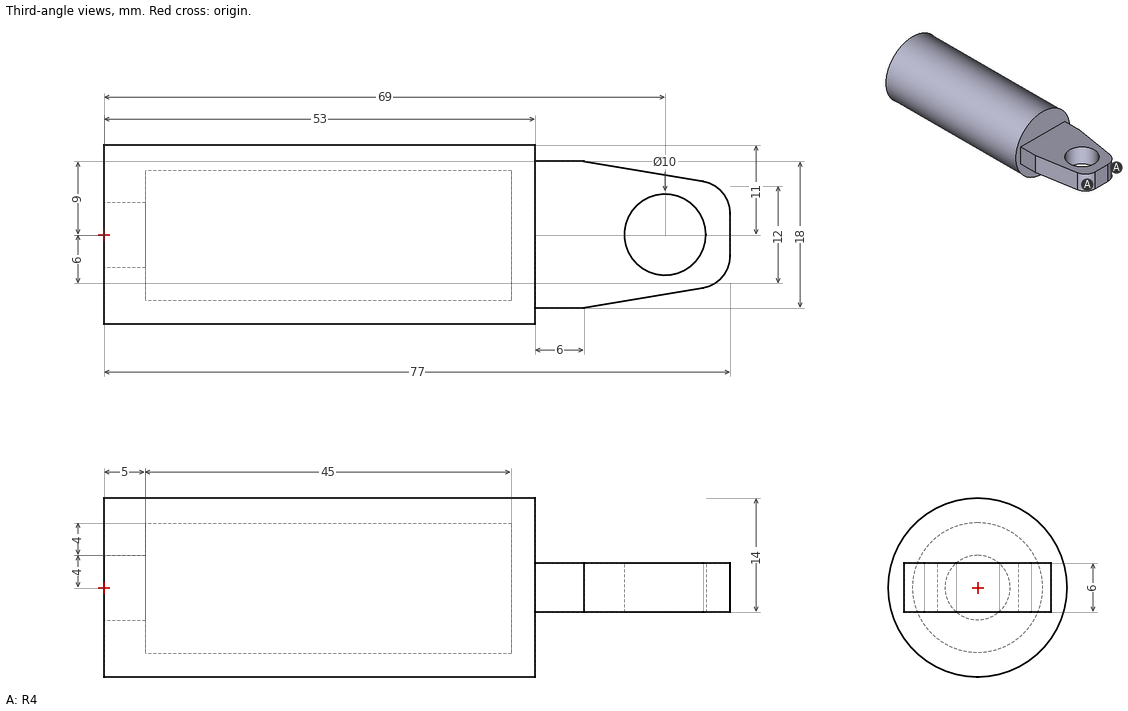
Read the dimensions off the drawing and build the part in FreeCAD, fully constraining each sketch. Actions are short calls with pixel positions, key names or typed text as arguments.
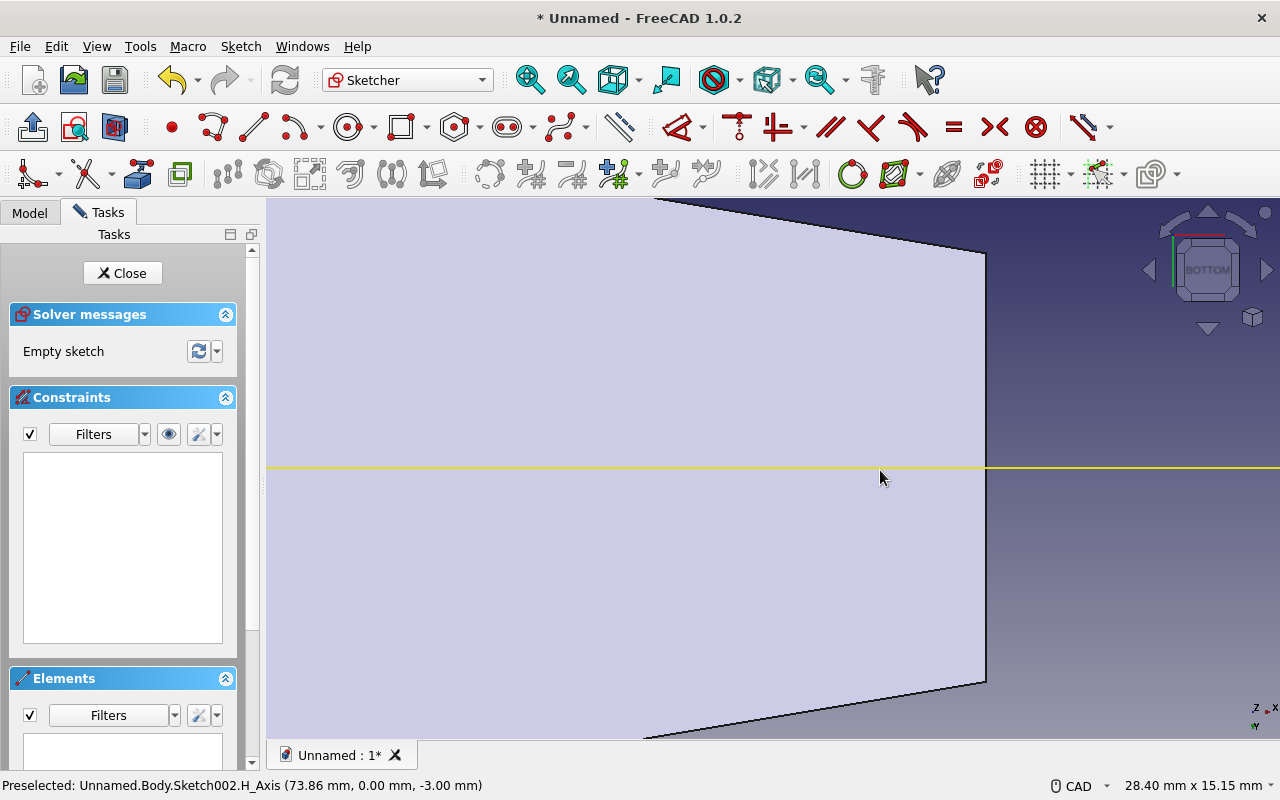
key(g)
key(c)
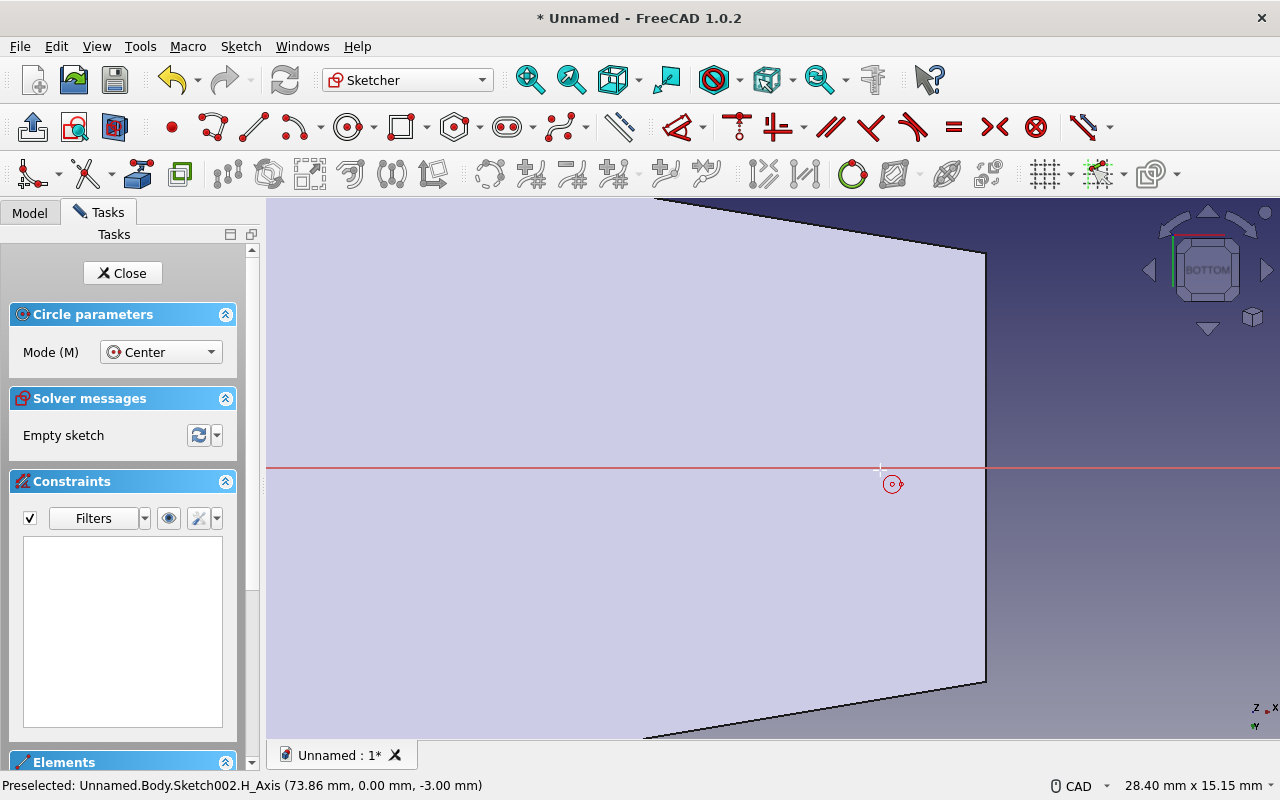
click(701, 468)
click(827, 341)
key(Escape)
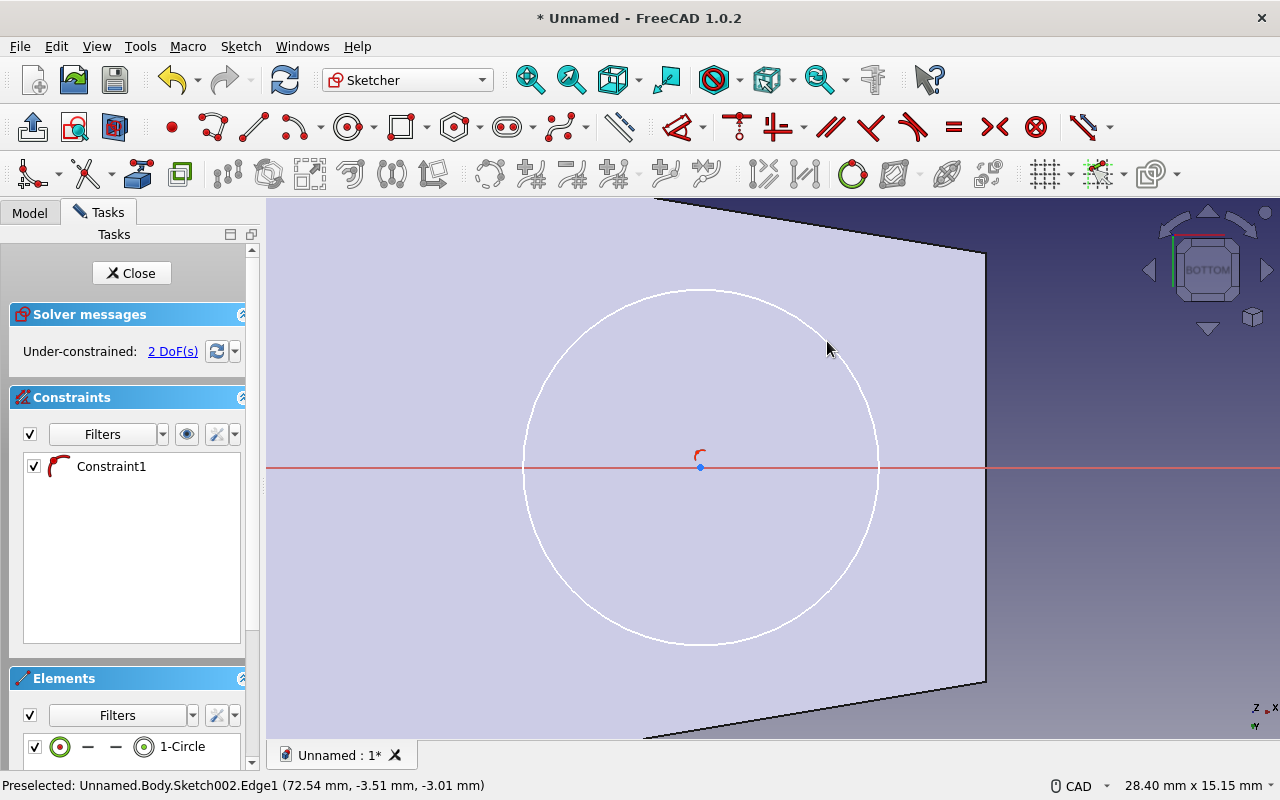
click(826, 341)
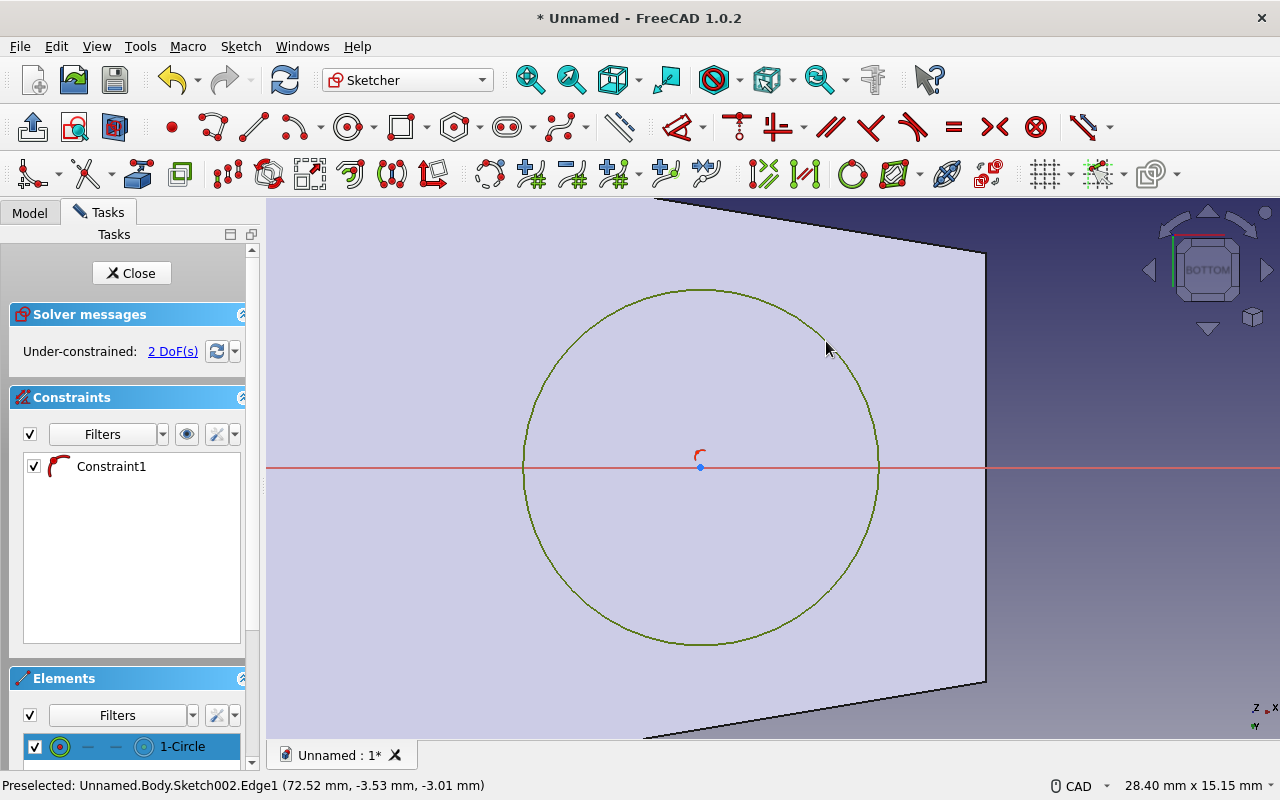
key(k)
key(o)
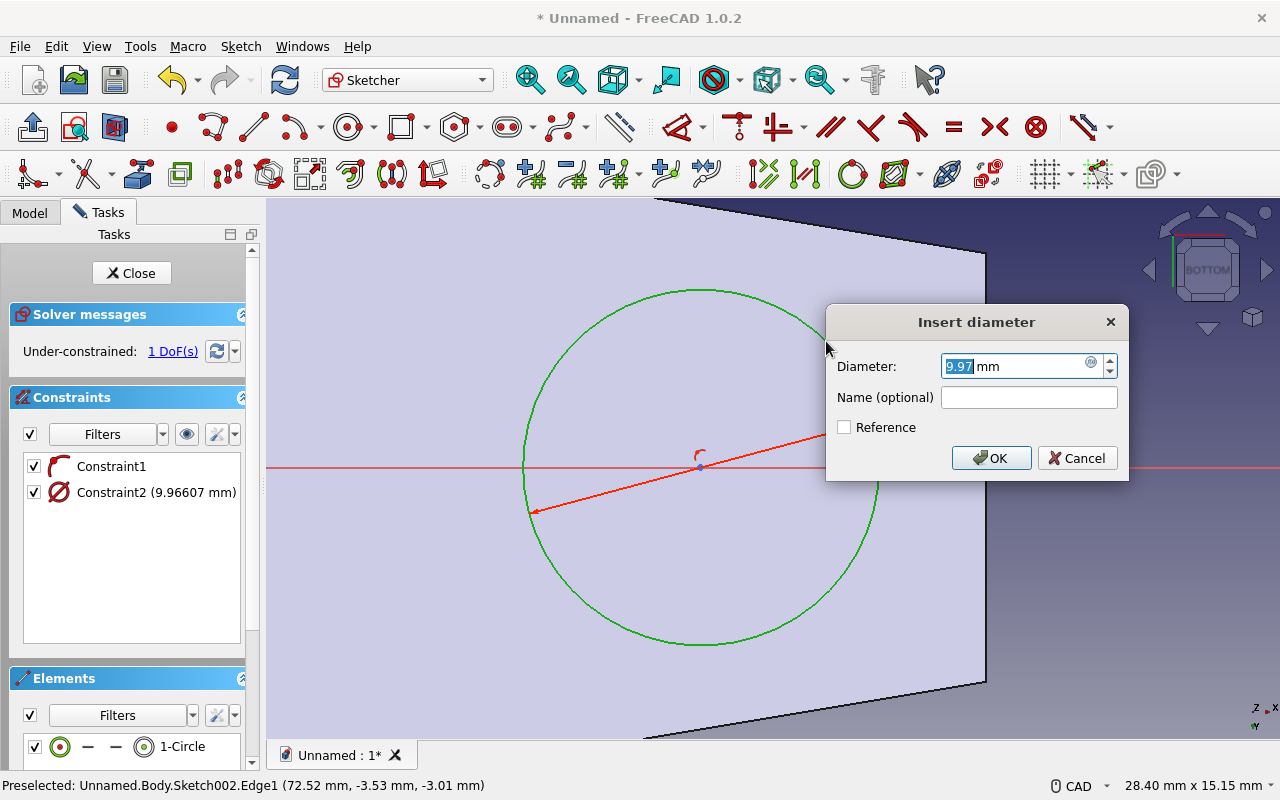
text(10)
key(Return)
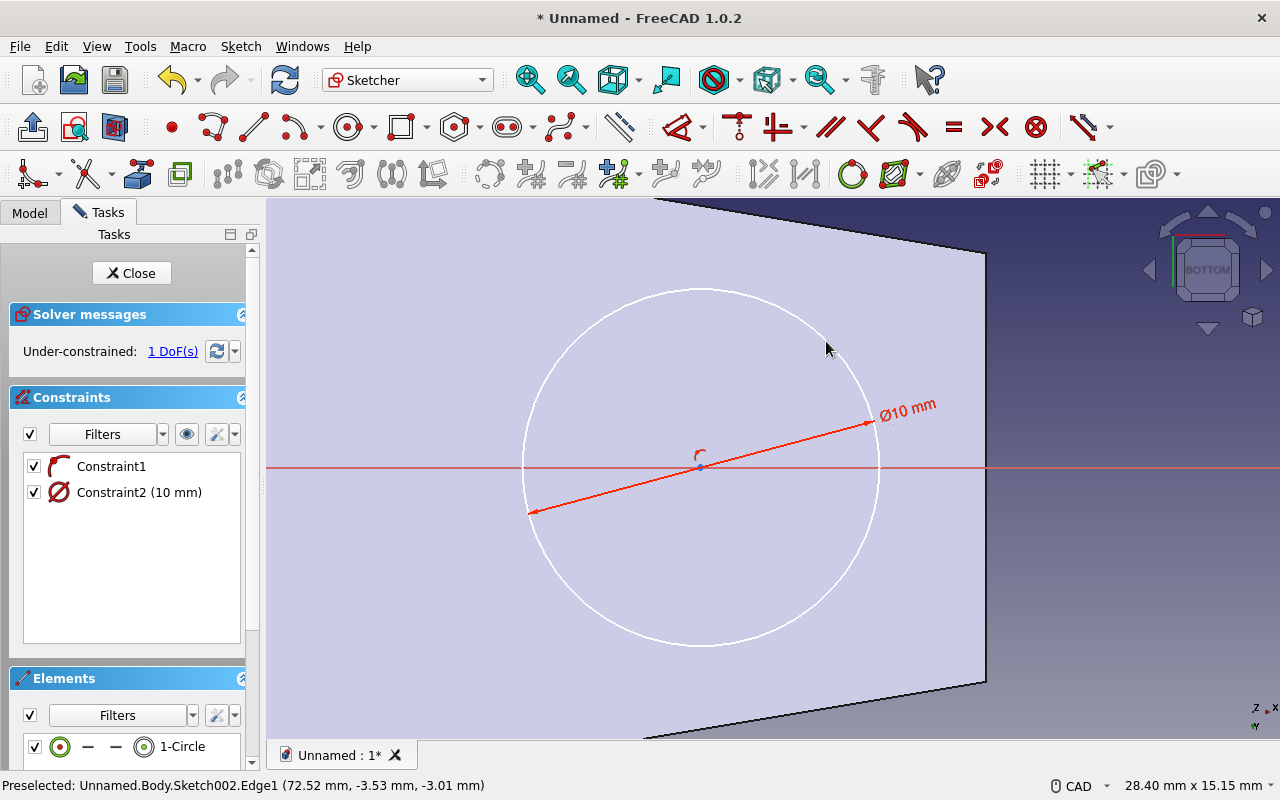
click(701, 468)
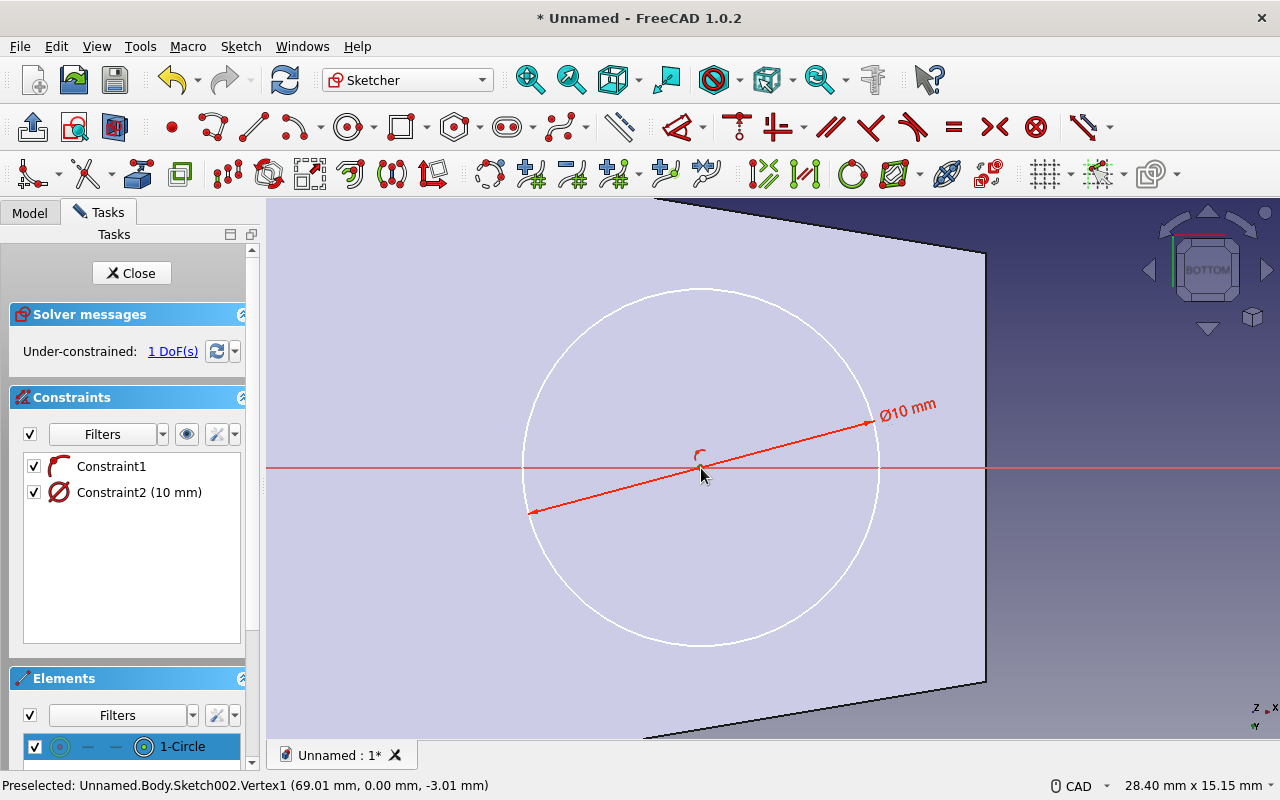
click(702, 128)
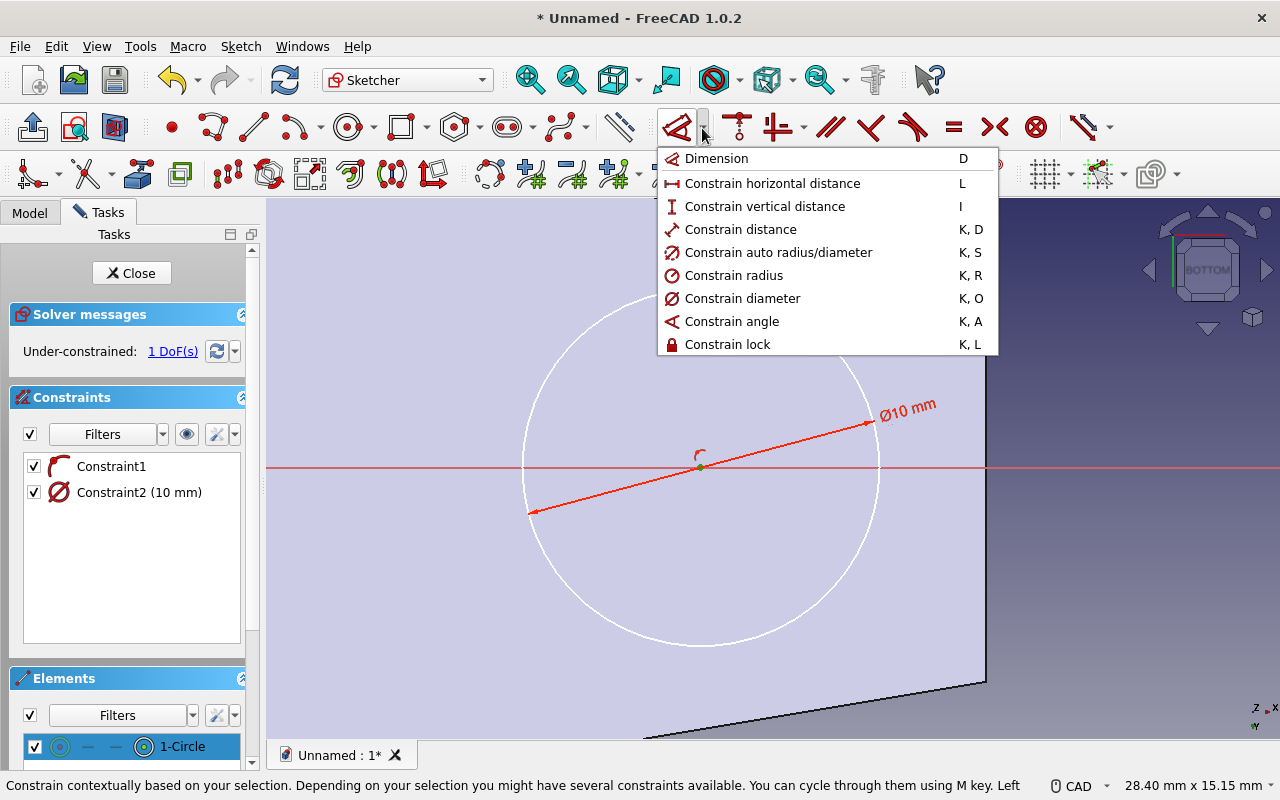
click(828, 184)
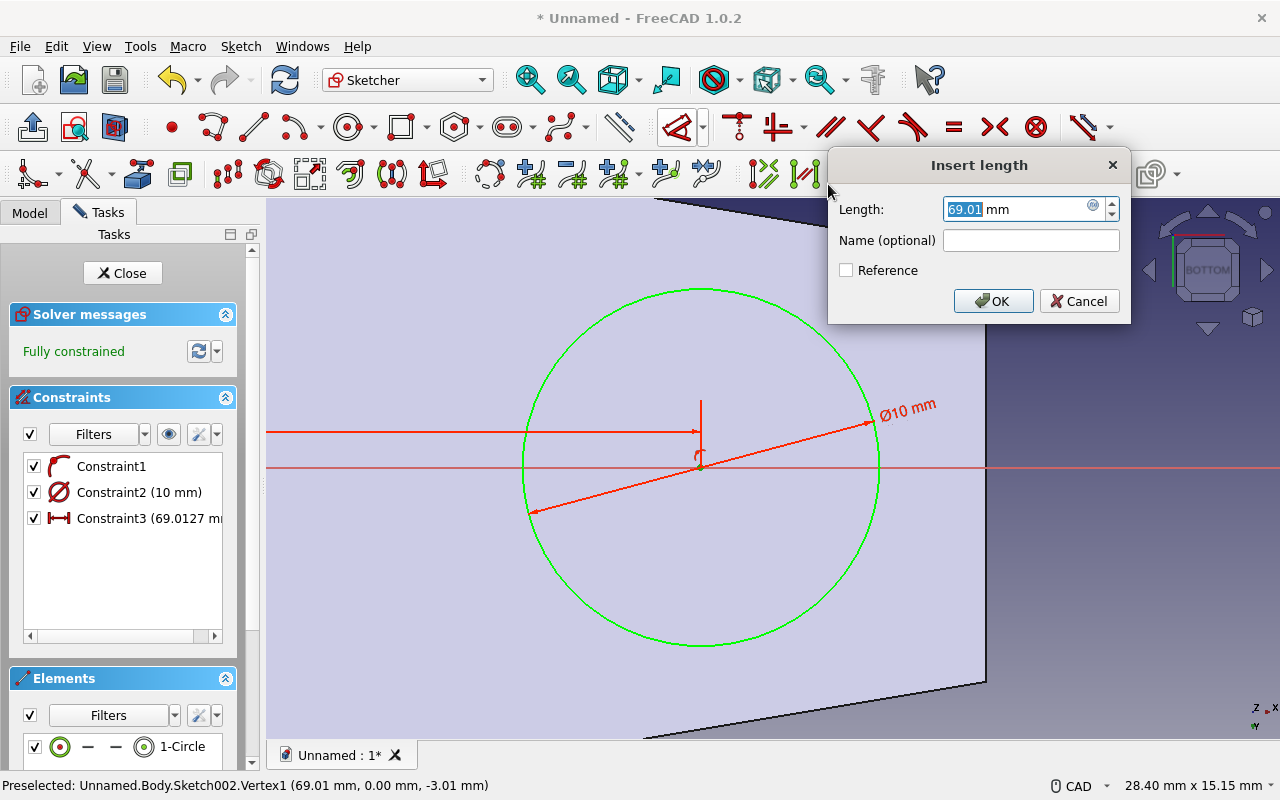
text(69)
key(Return)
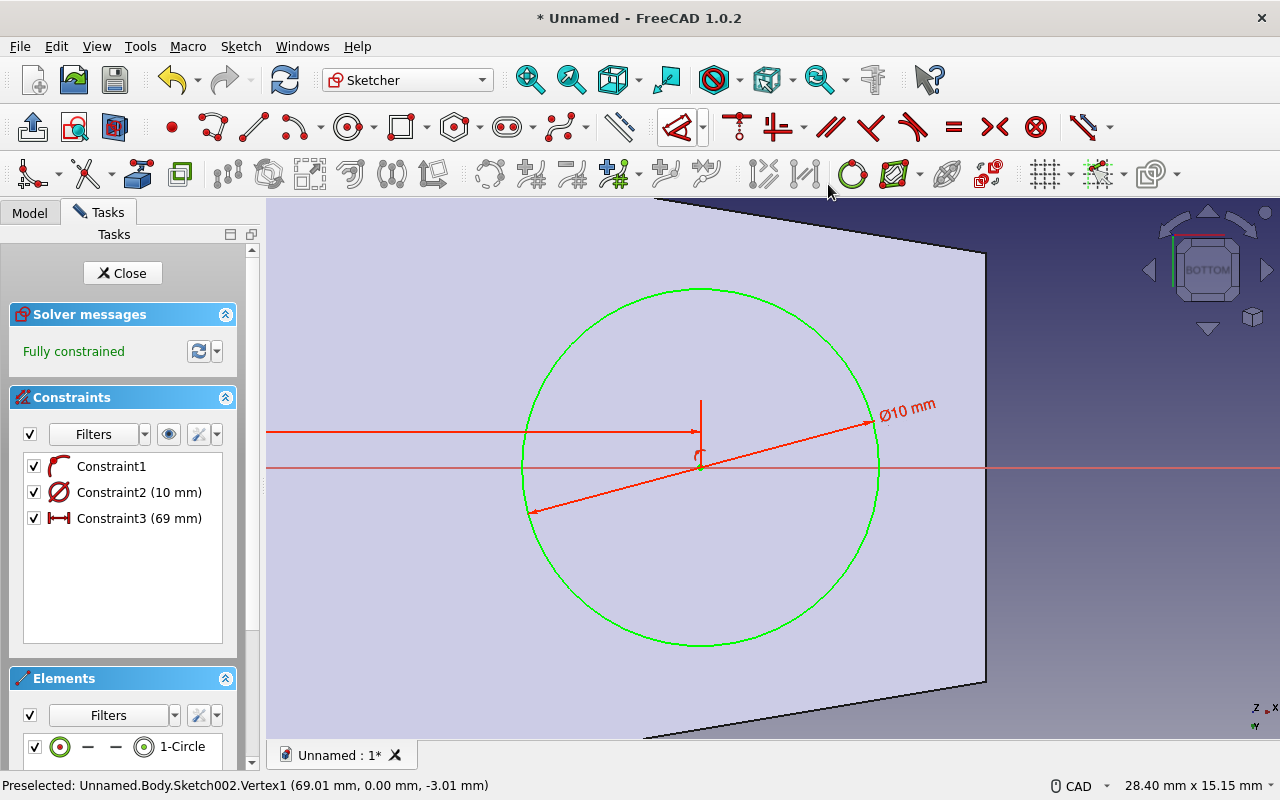
click(123, 273)